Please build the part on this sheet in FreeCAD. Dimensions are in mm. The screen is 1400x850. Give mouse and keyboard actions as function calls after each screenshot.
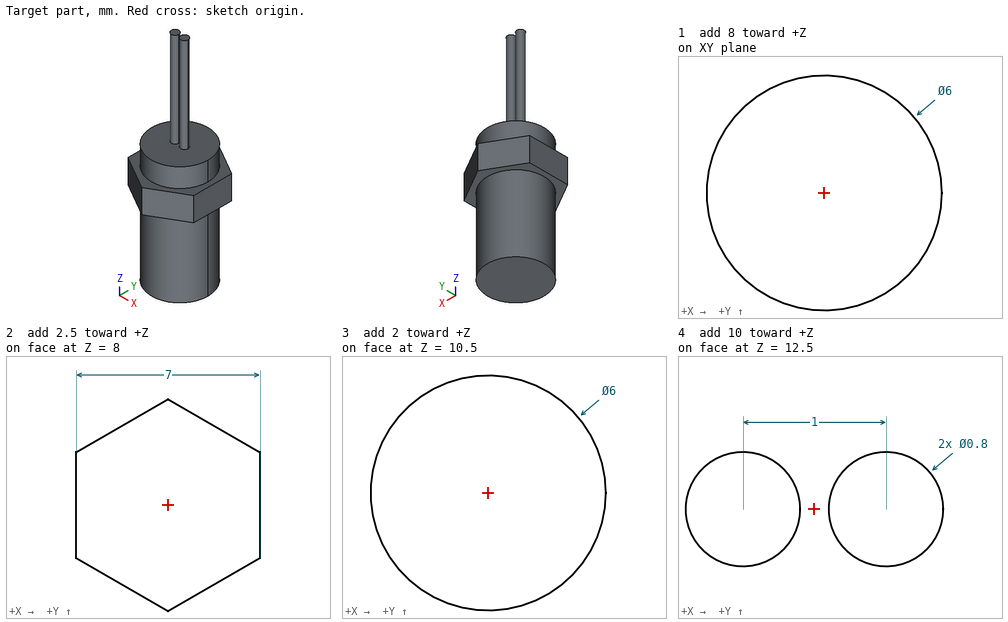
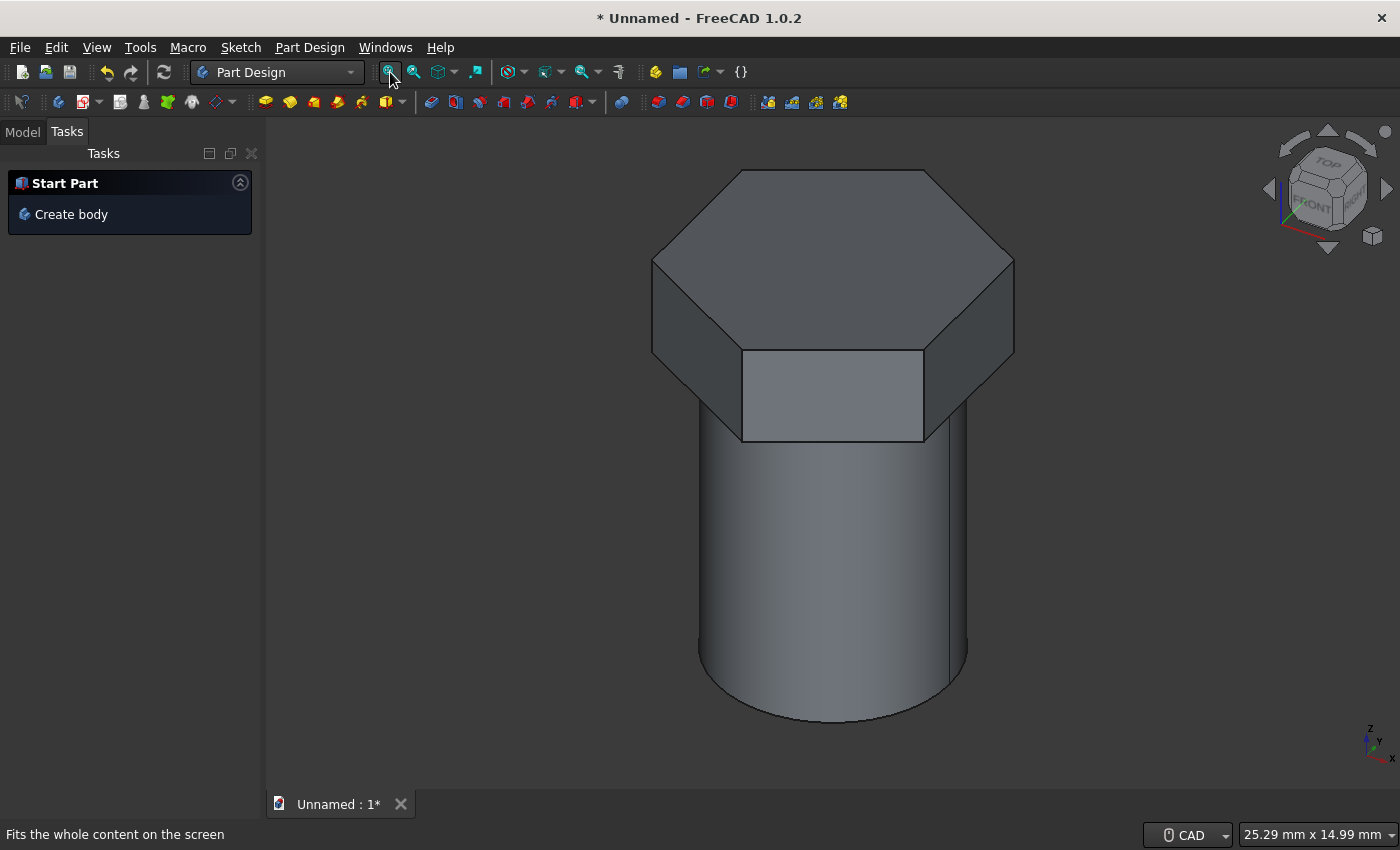
click(833, 259)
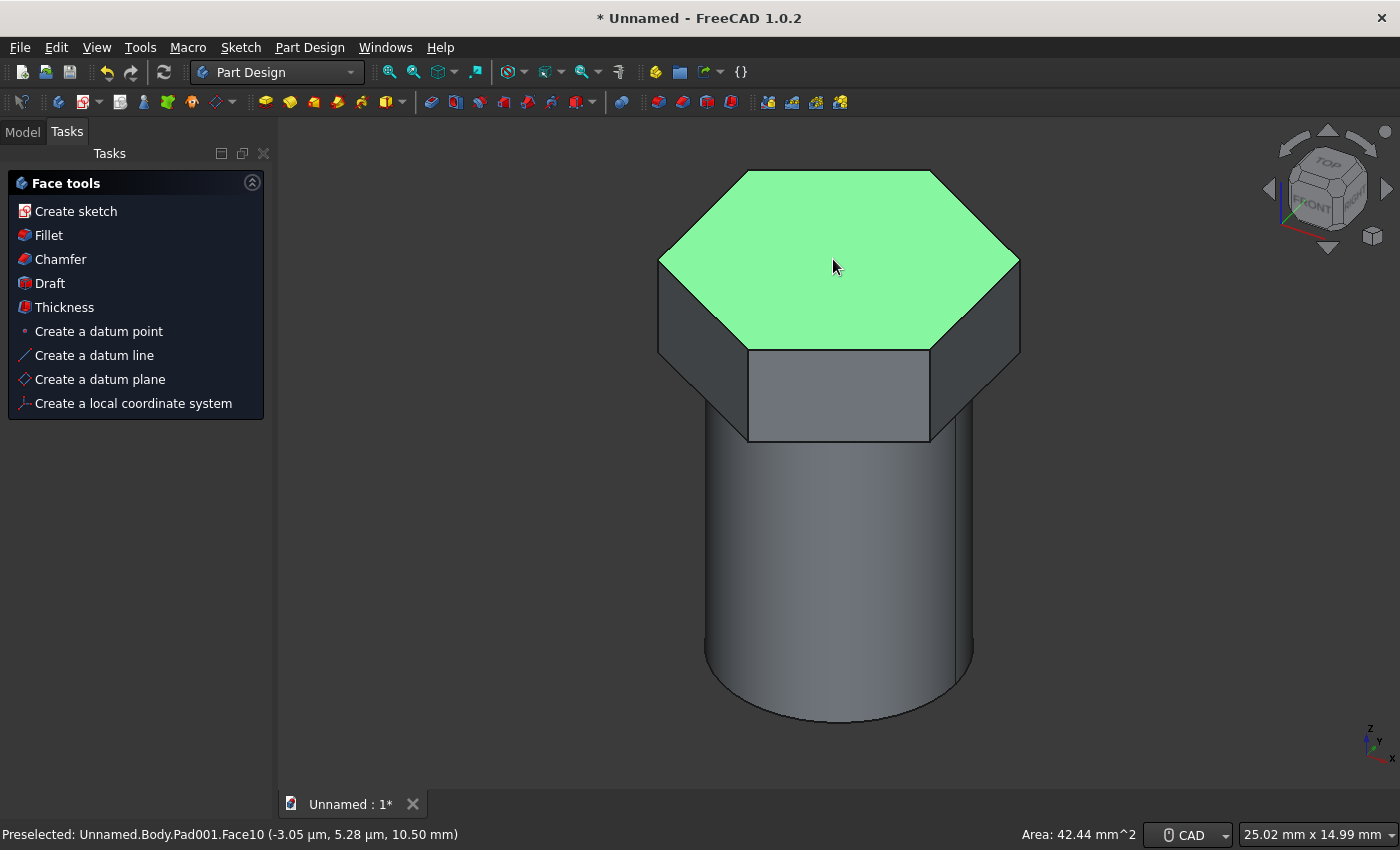
click(84, 102)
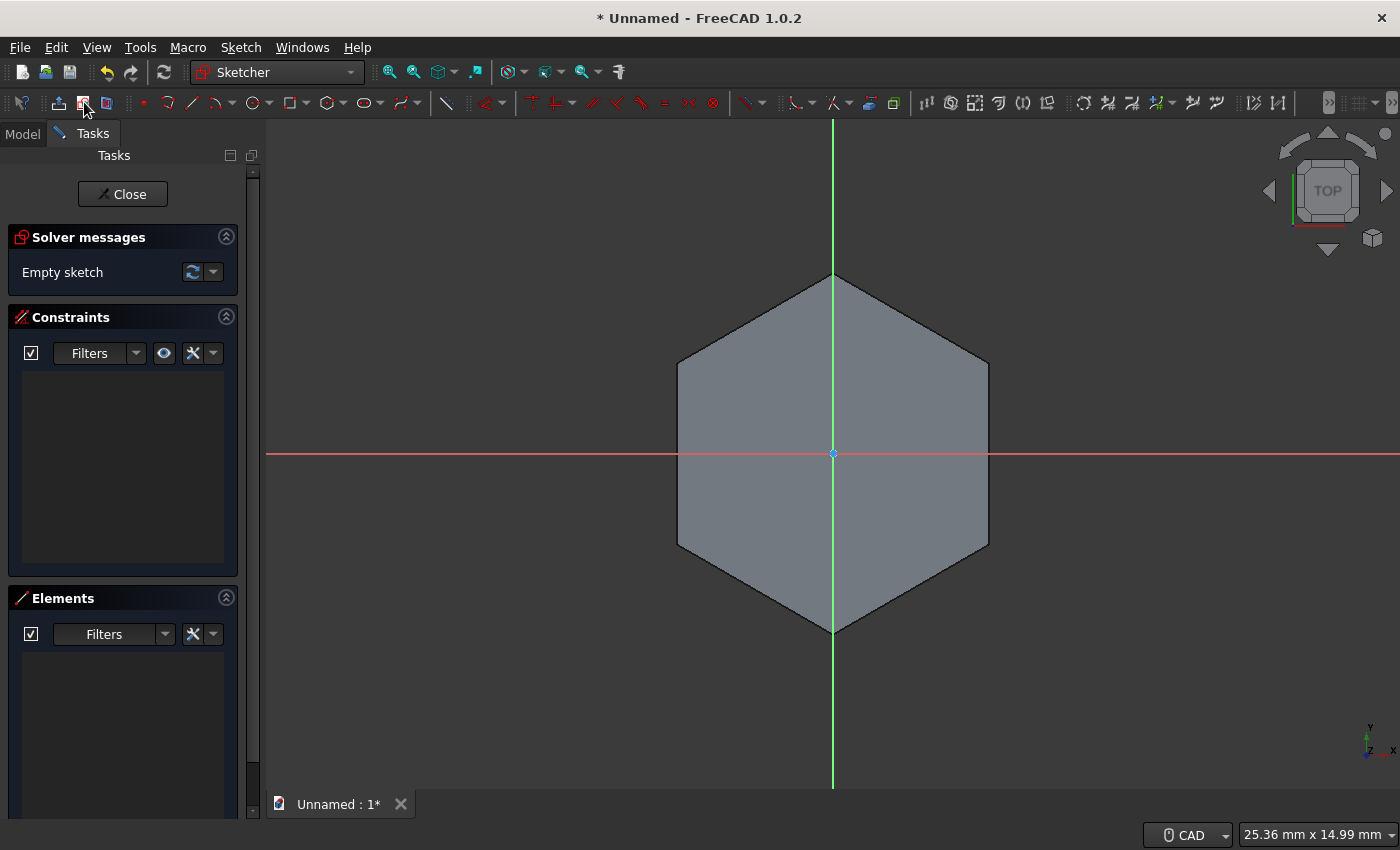
scroll(972, 454, up, 2)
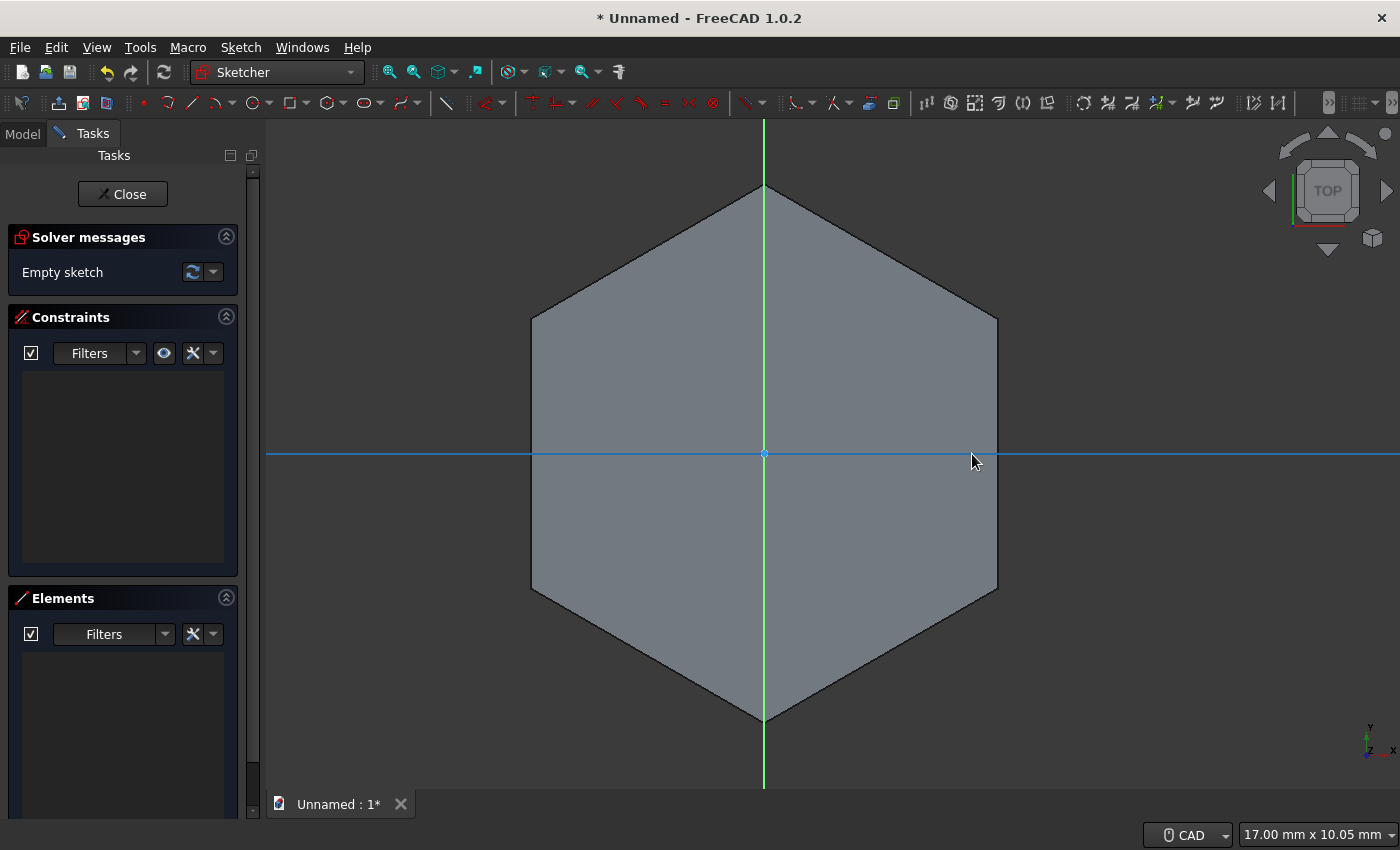
key(g)
key(c)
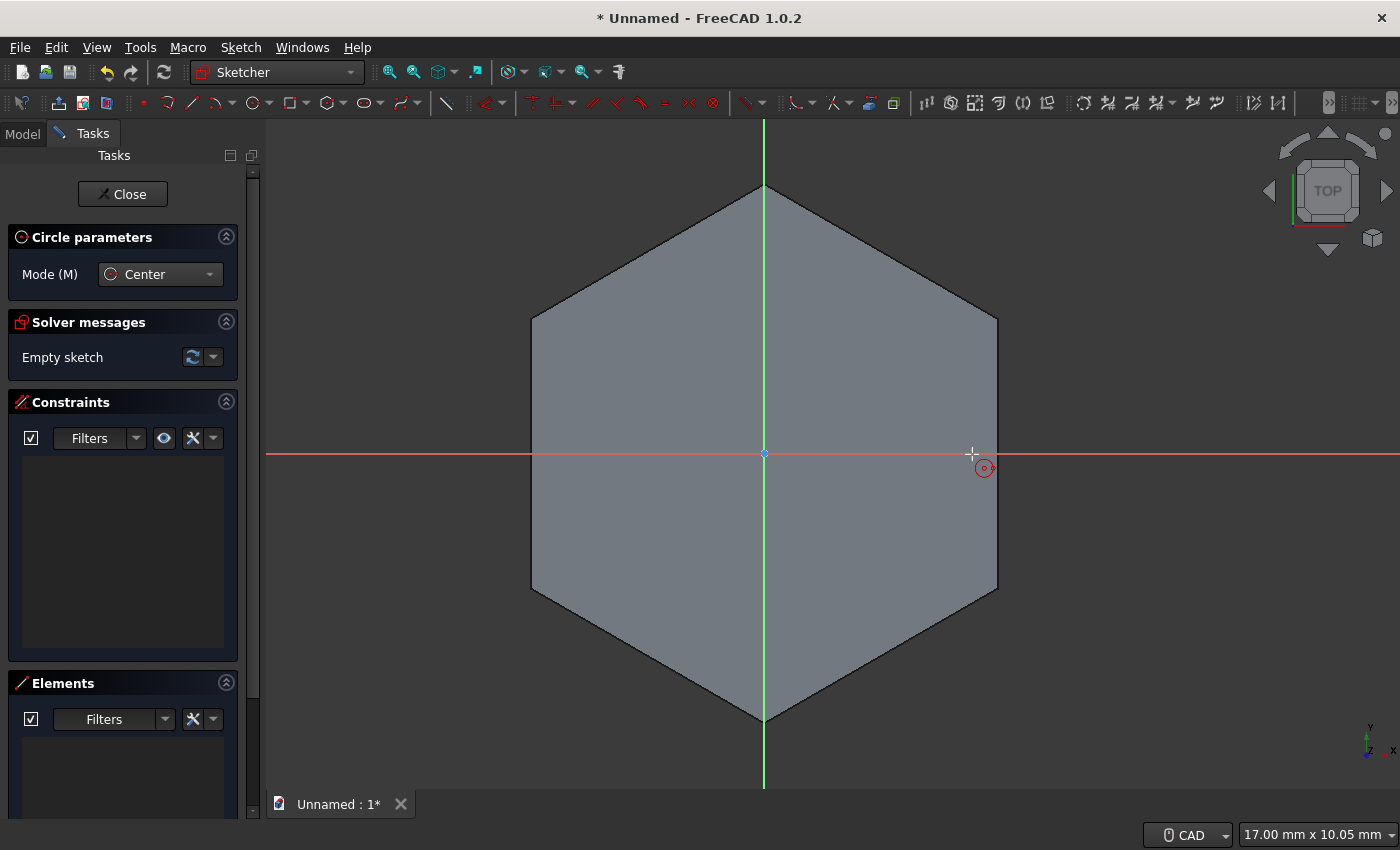
click(764, 454)
move(906, 312)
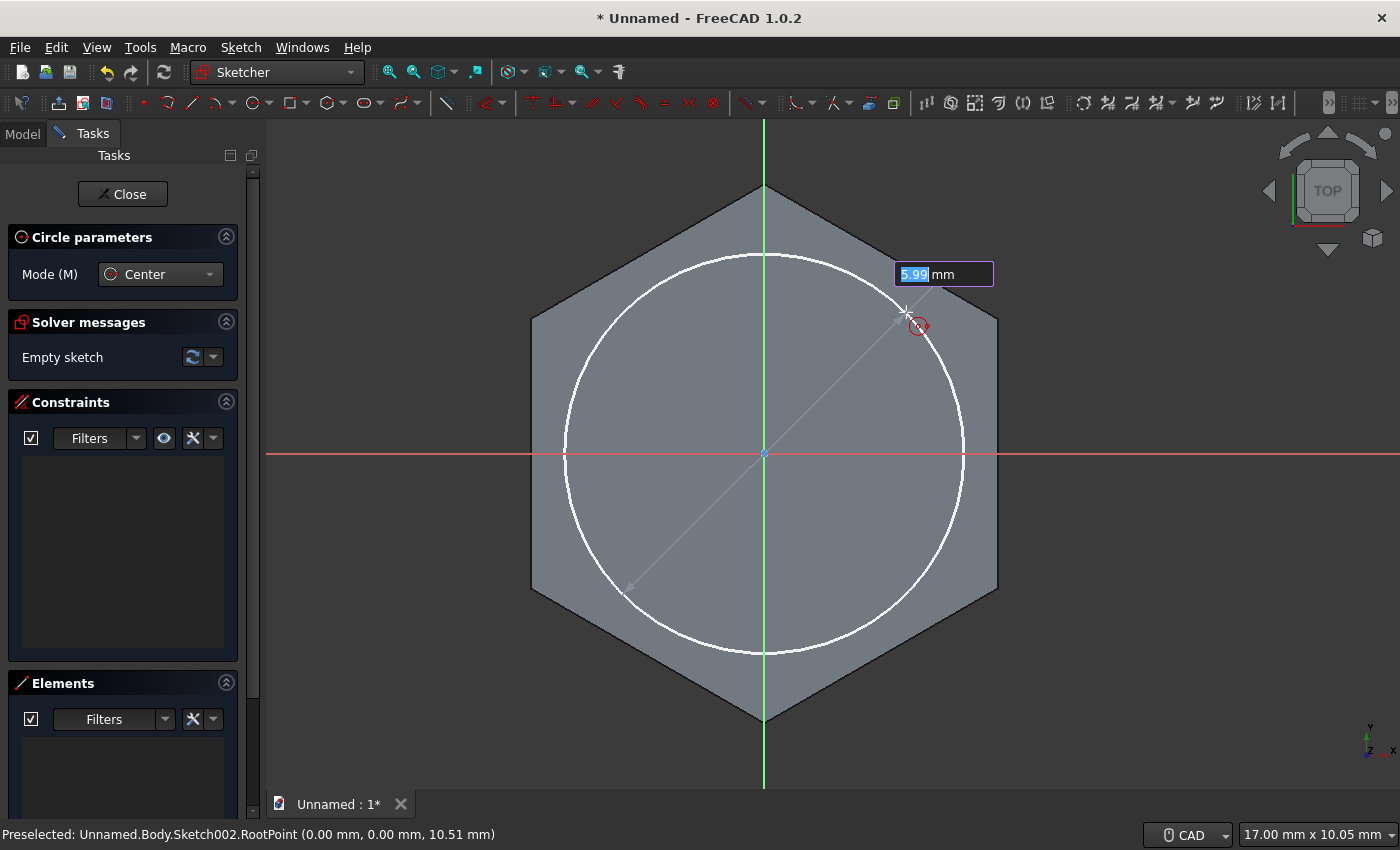
text(6)
key(Return)
key(Escape)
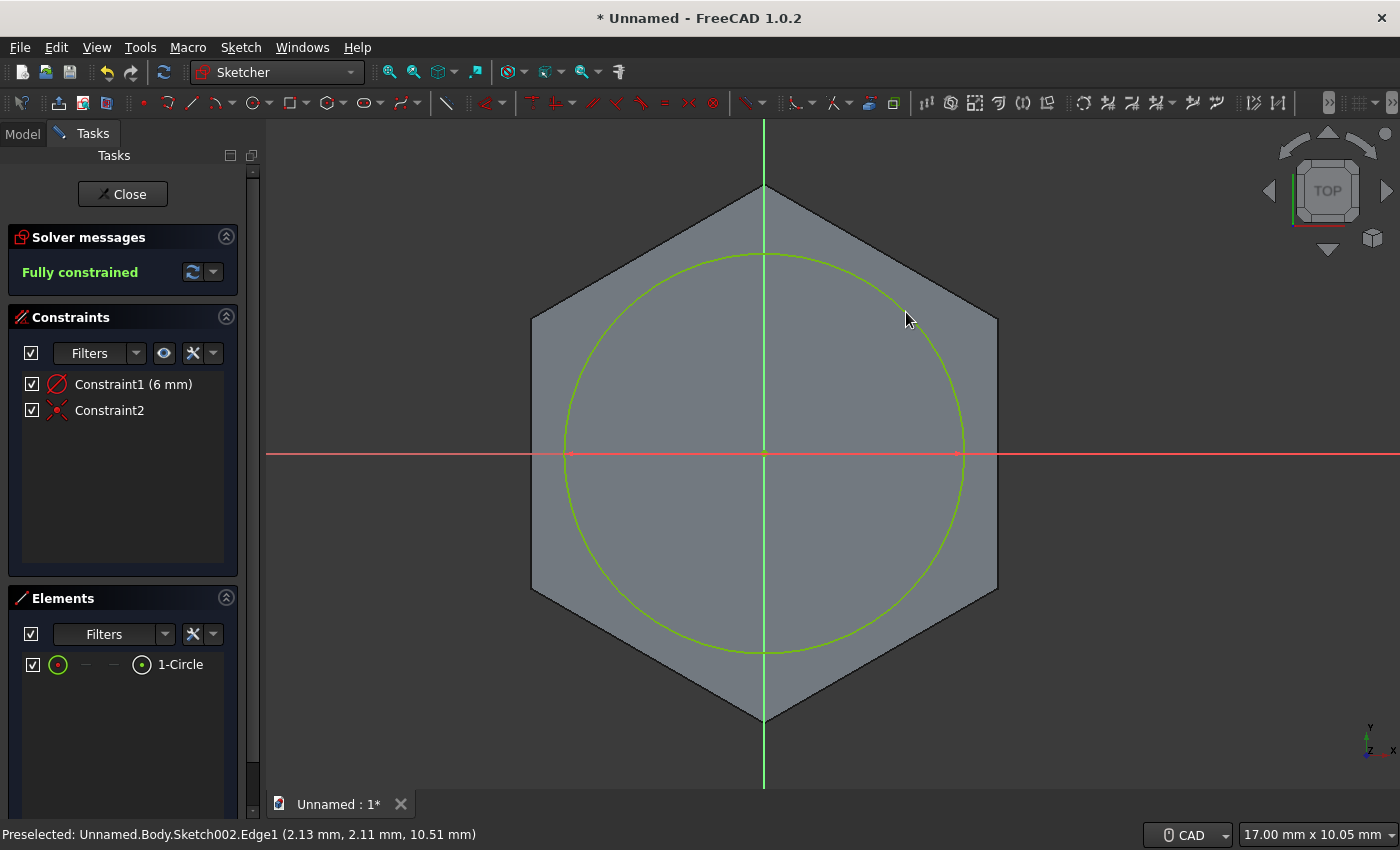
click(123, 194)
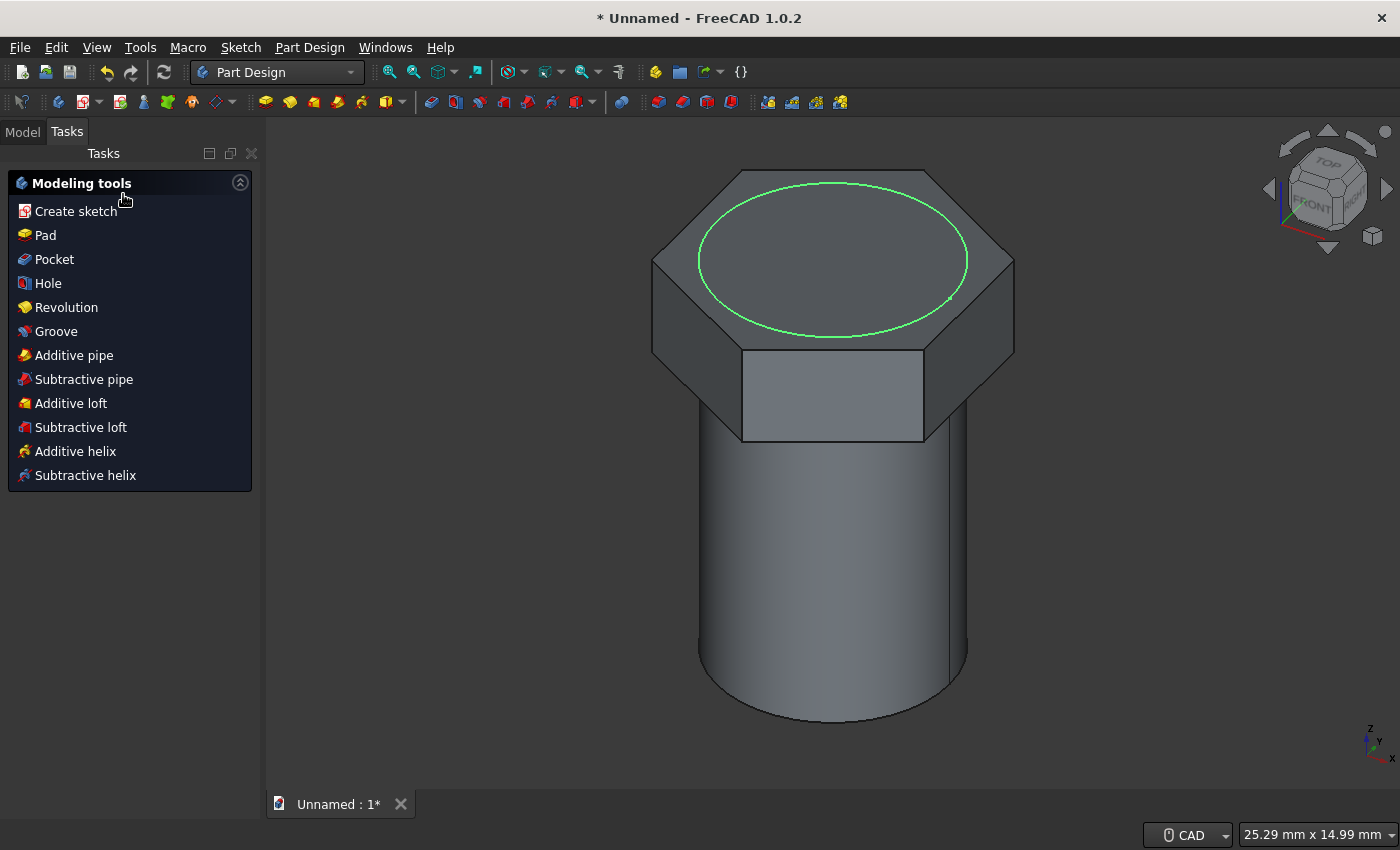
click(266, 102)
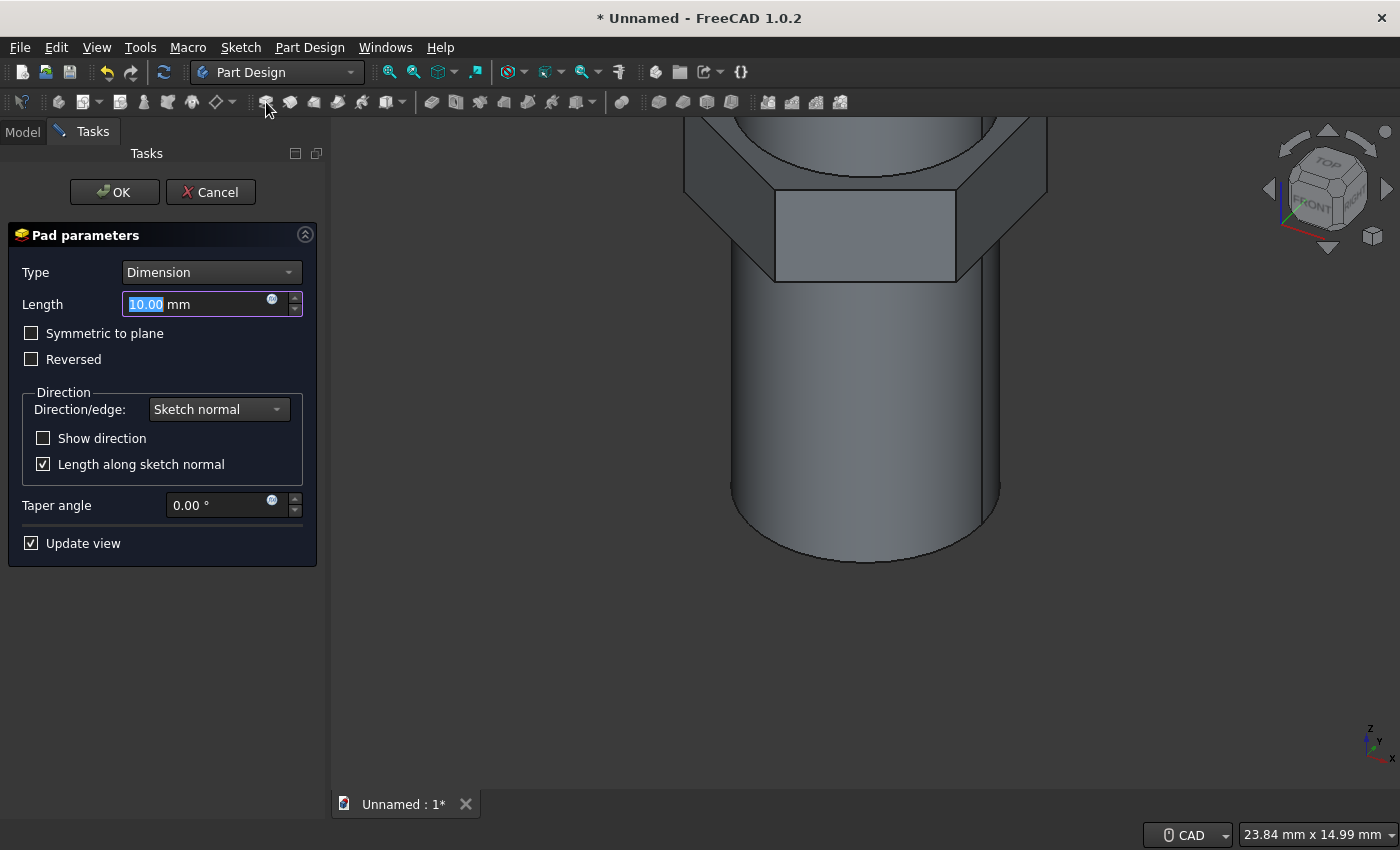
text(2)
key(Tab)